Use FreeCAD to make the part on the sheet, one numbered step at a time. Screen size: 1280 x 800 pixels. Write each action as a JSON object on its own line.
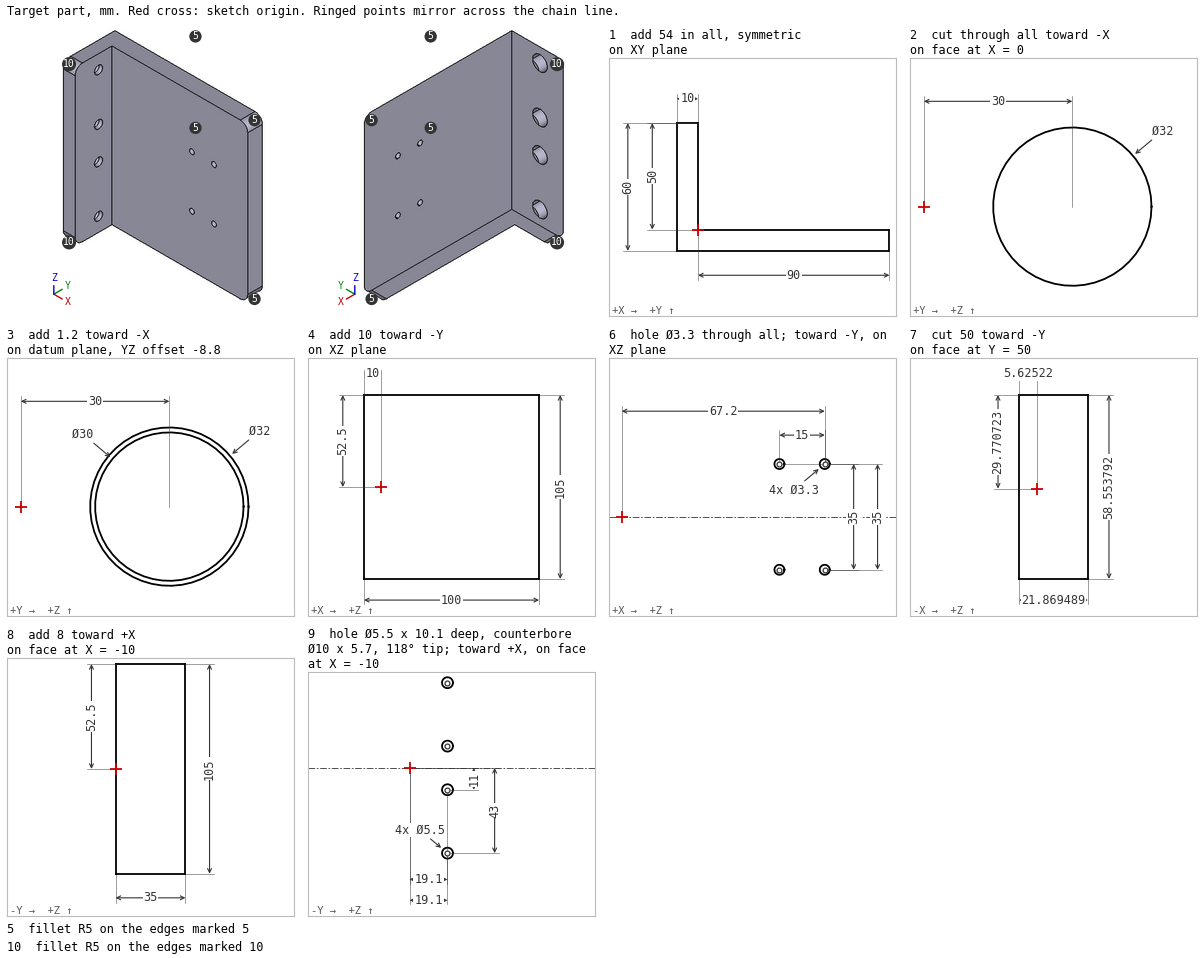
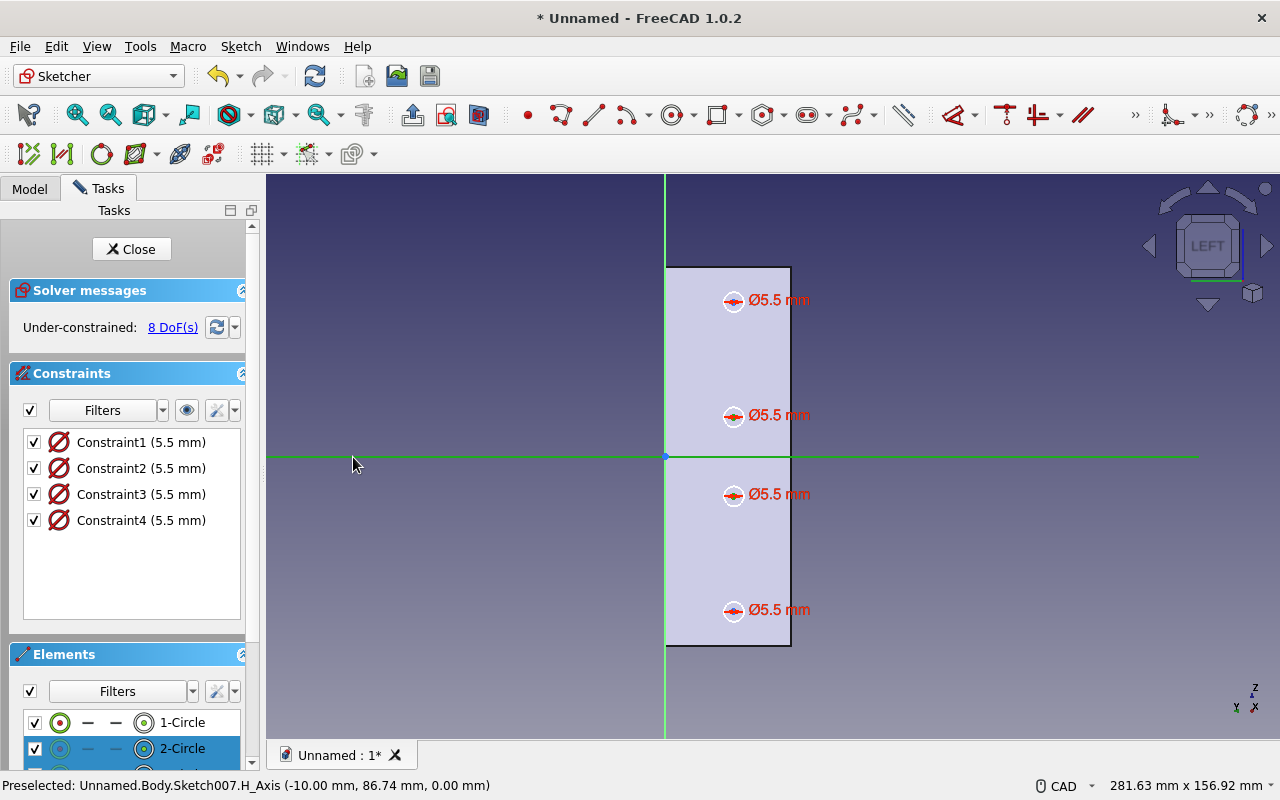
{"action": "key", "text": "s"}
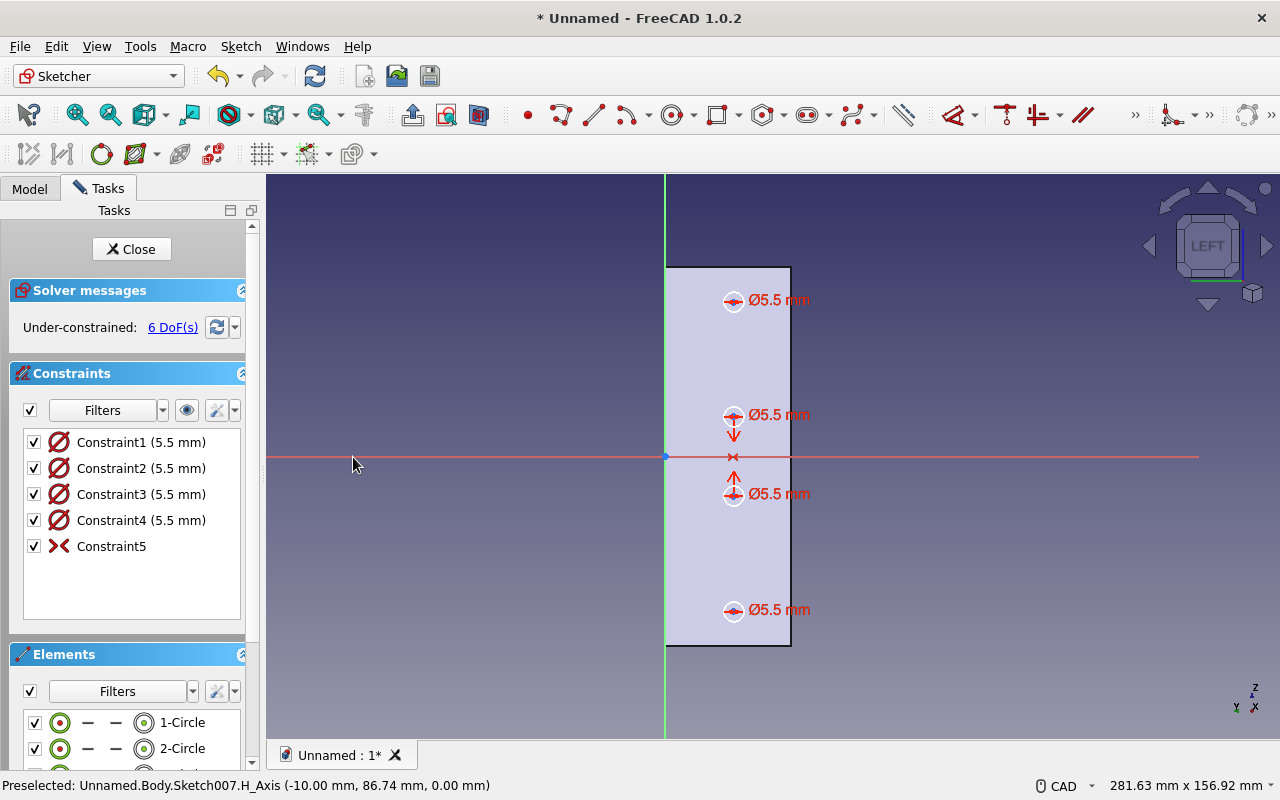
{"action": "left_click", "coordinate": [734, 612]}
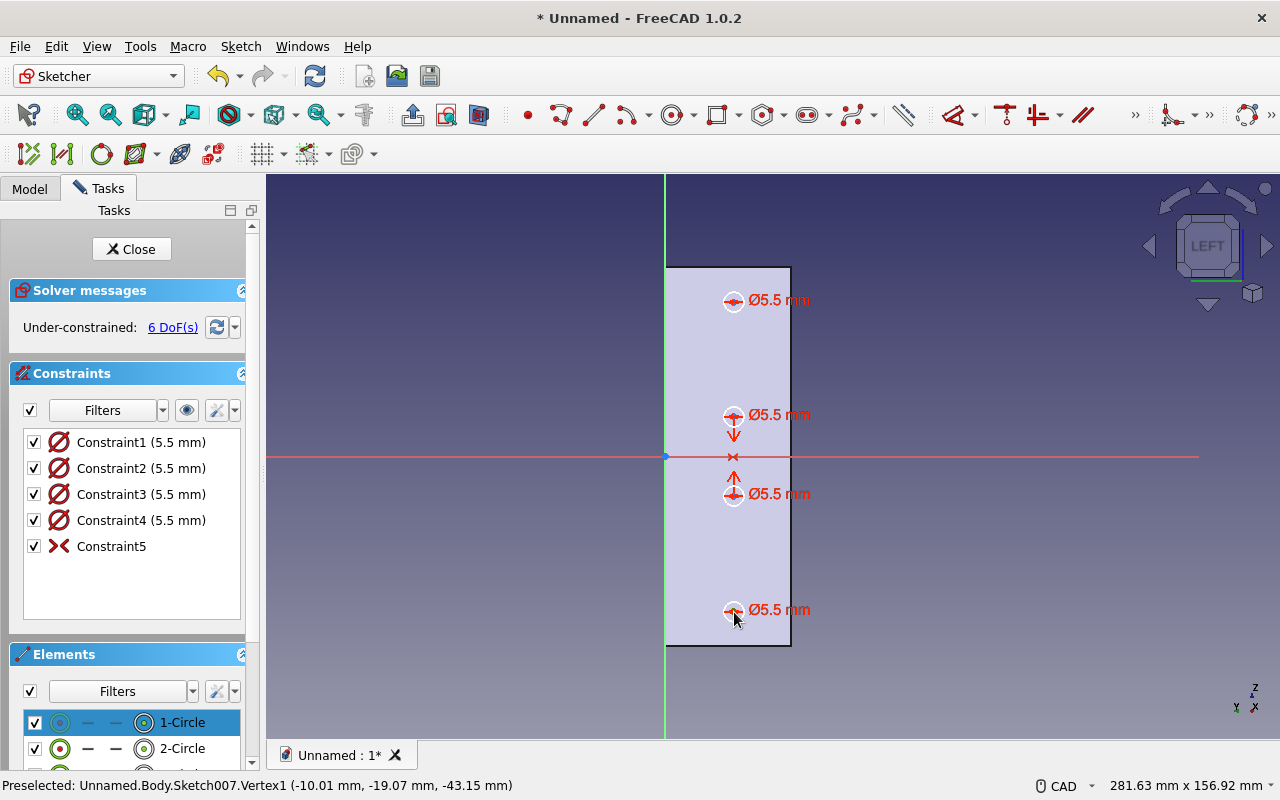
{"action": "left_click", "coordinate": [734, 302]}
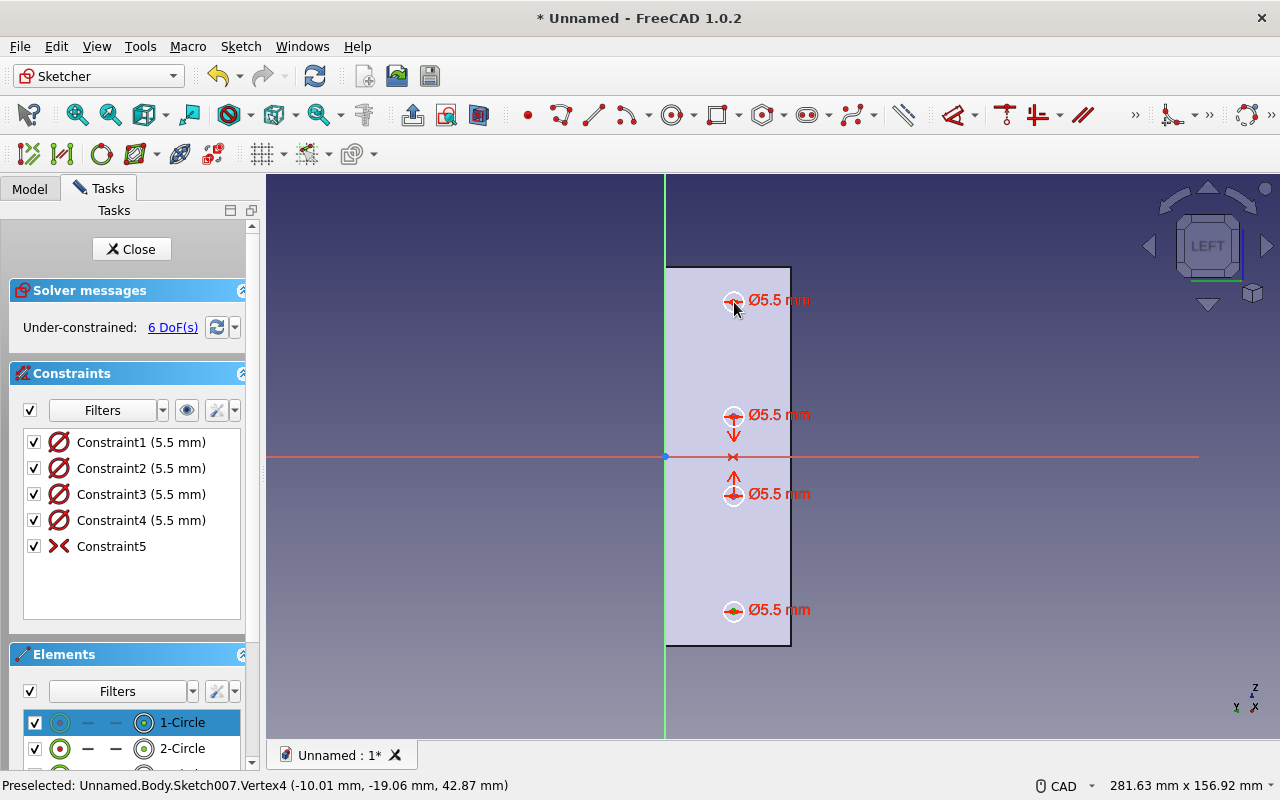
{"action": "left_click", "coordinate": [353, 457]}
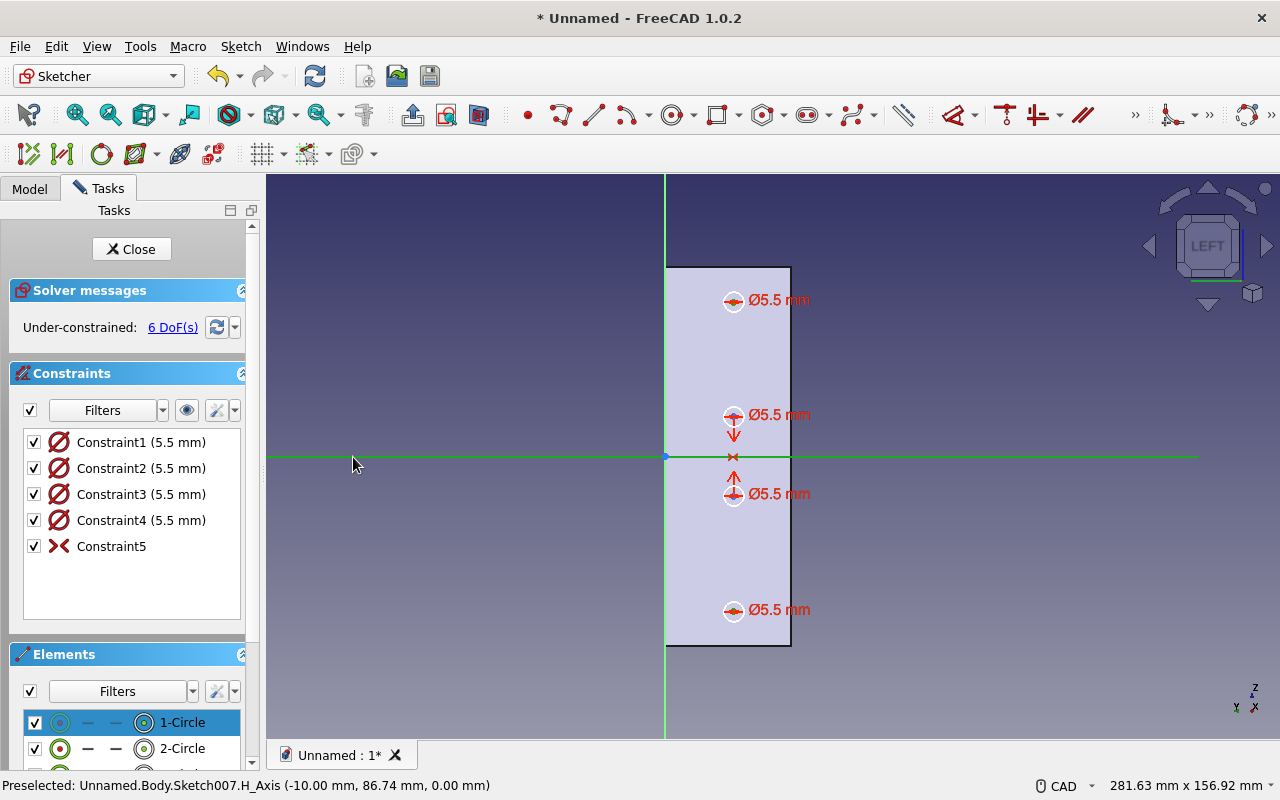
{"action": "key", "text": "s"}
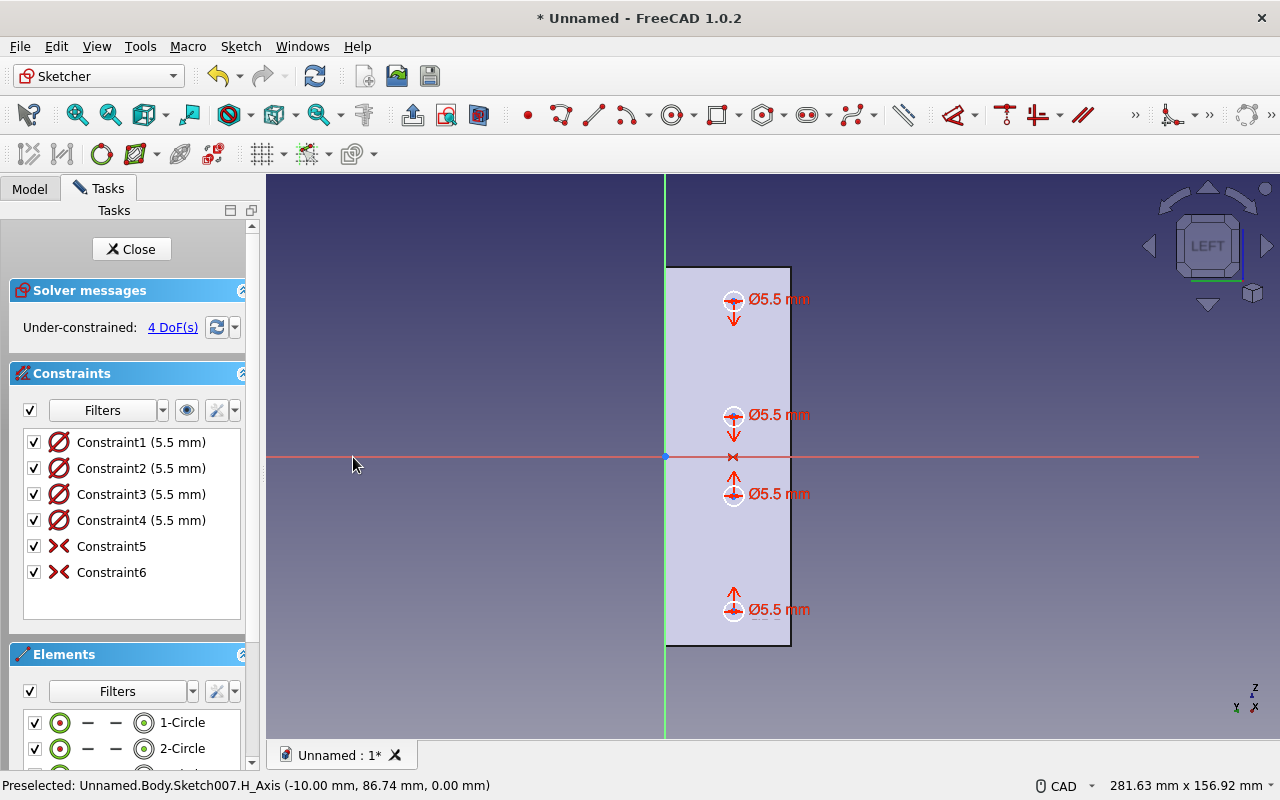
{"action": "left_click", "coordinate": [952, 116]}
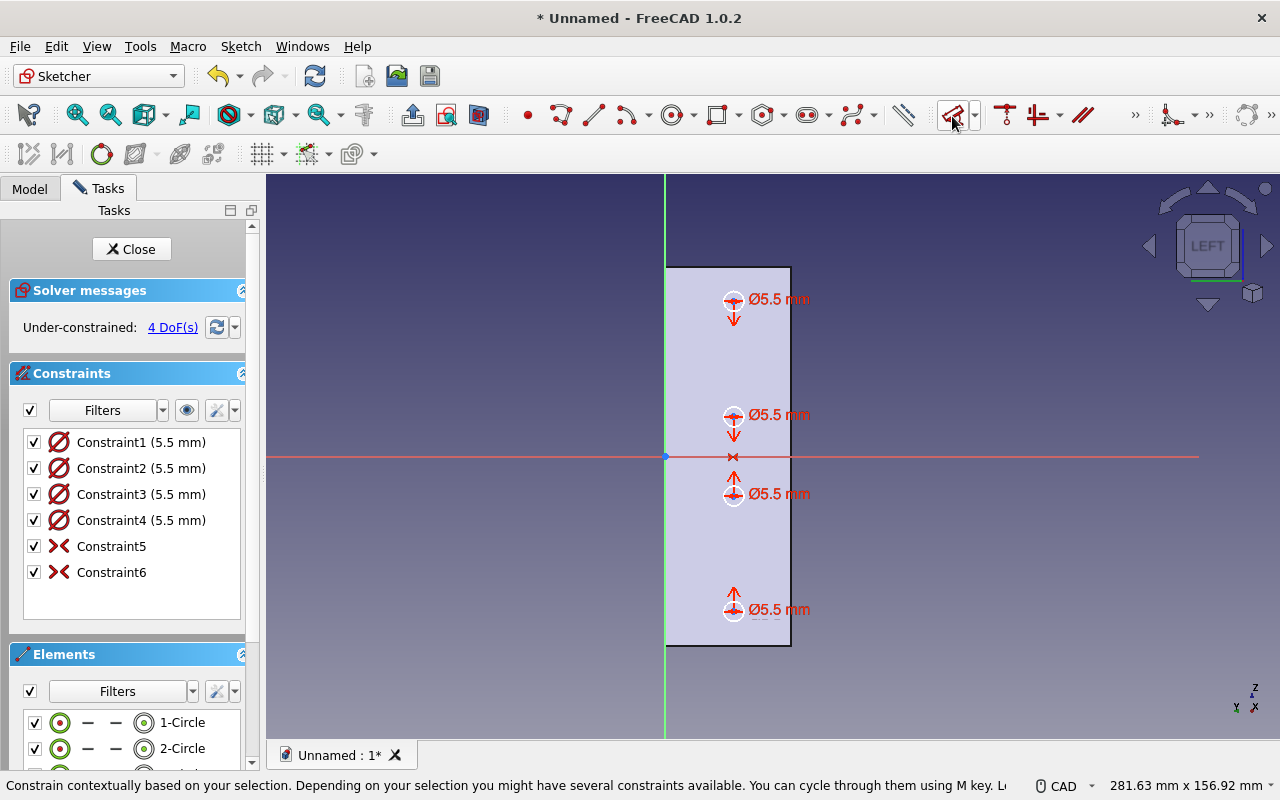
{"action": "left_click", "coordinate": [734, 612]}
{"action": "left_click", "coordinate": [631, 534]}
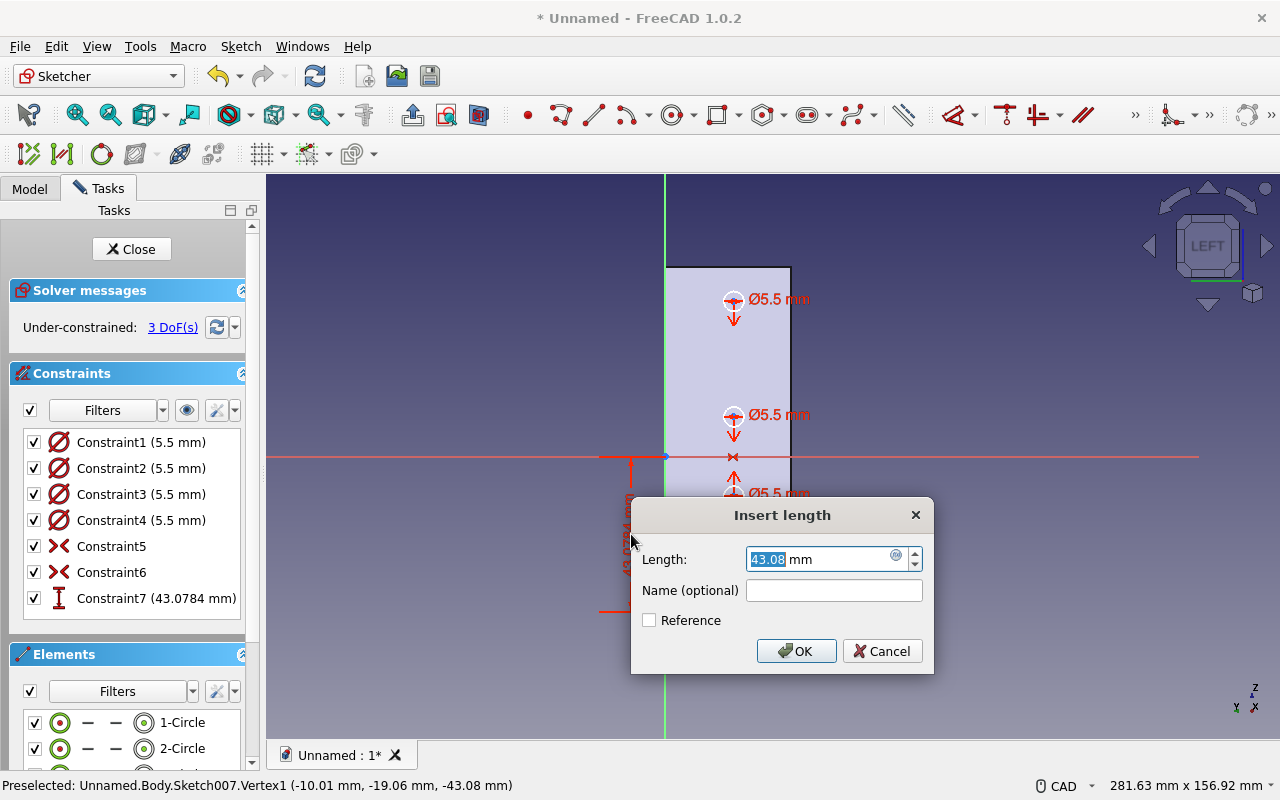
{"action": "type", "text": "43"}
{"action": "key", "text": "Return"}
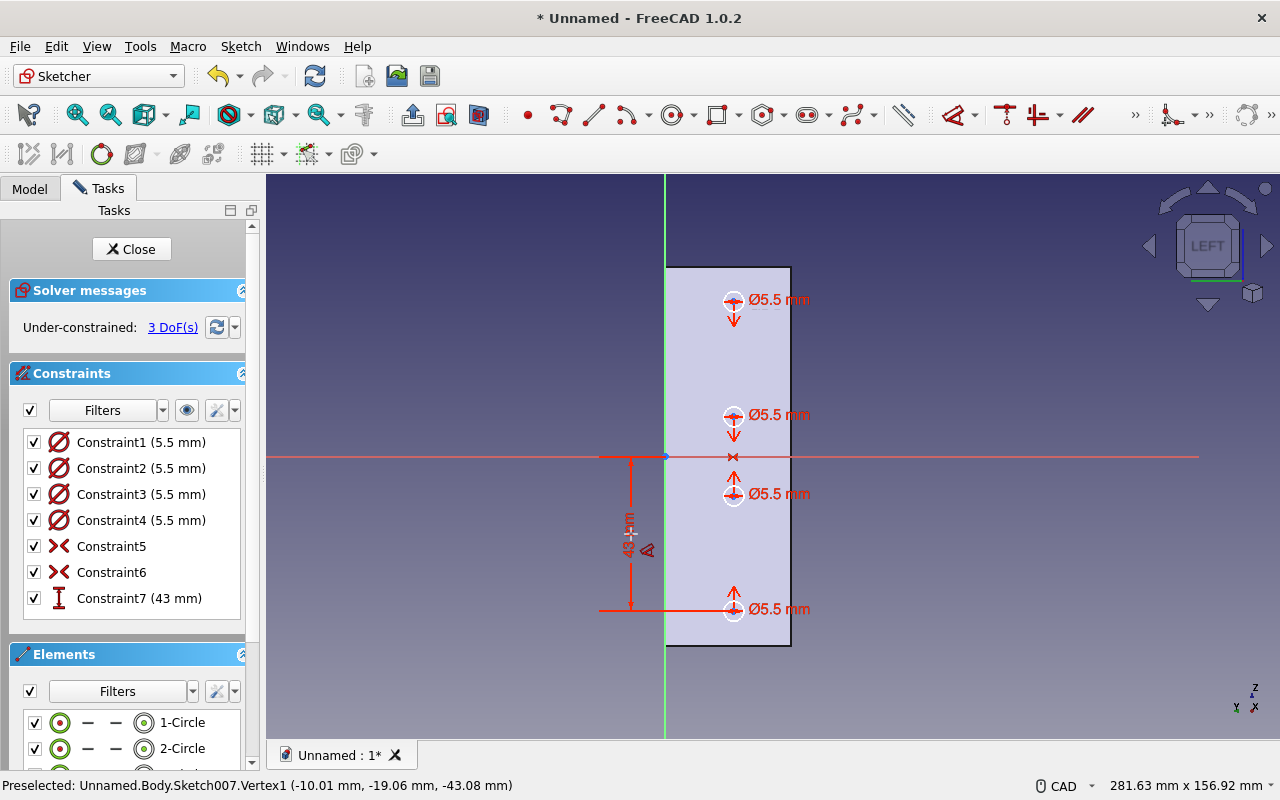
{"action": "left_click", "coordinate": [734, 496]}
{"action": "left_click", "coordinate": [631, 476]}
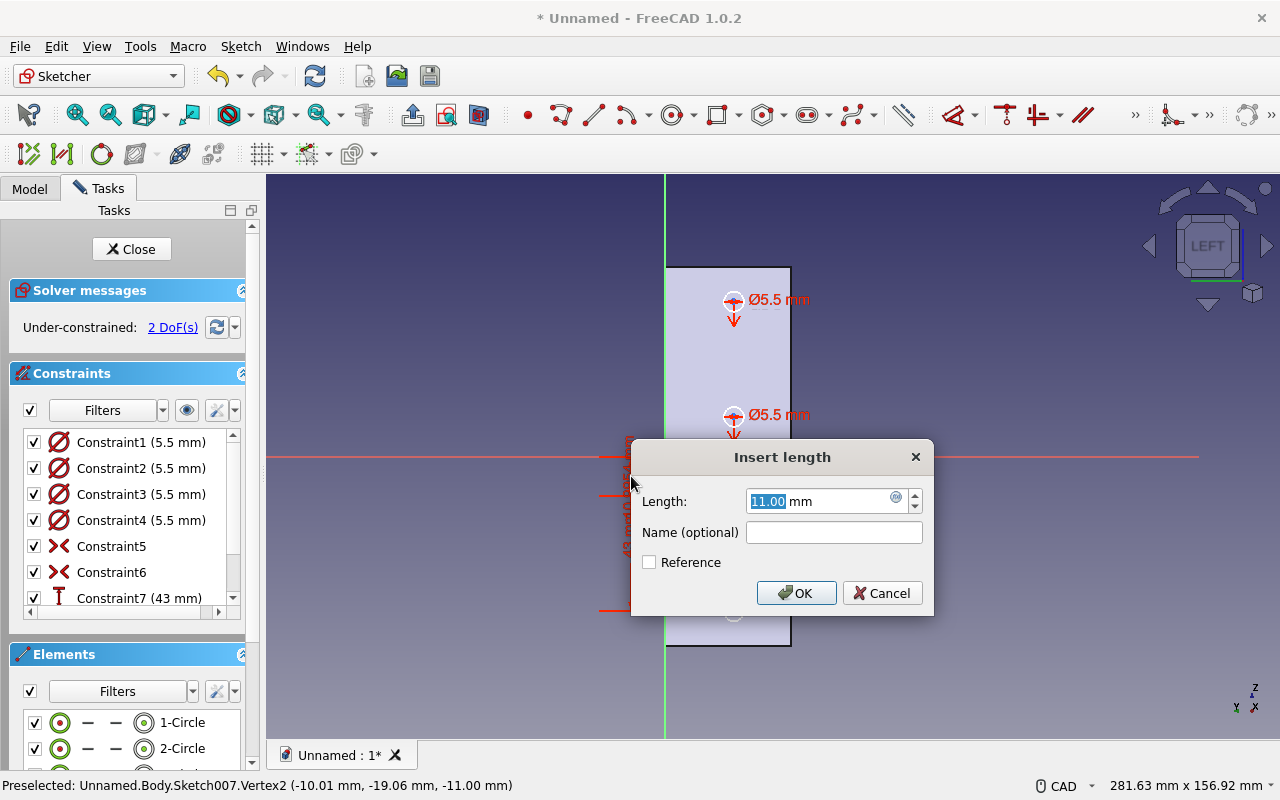
{"action": "type", "text": "11"}
{"action": "key", "text": "Return"}